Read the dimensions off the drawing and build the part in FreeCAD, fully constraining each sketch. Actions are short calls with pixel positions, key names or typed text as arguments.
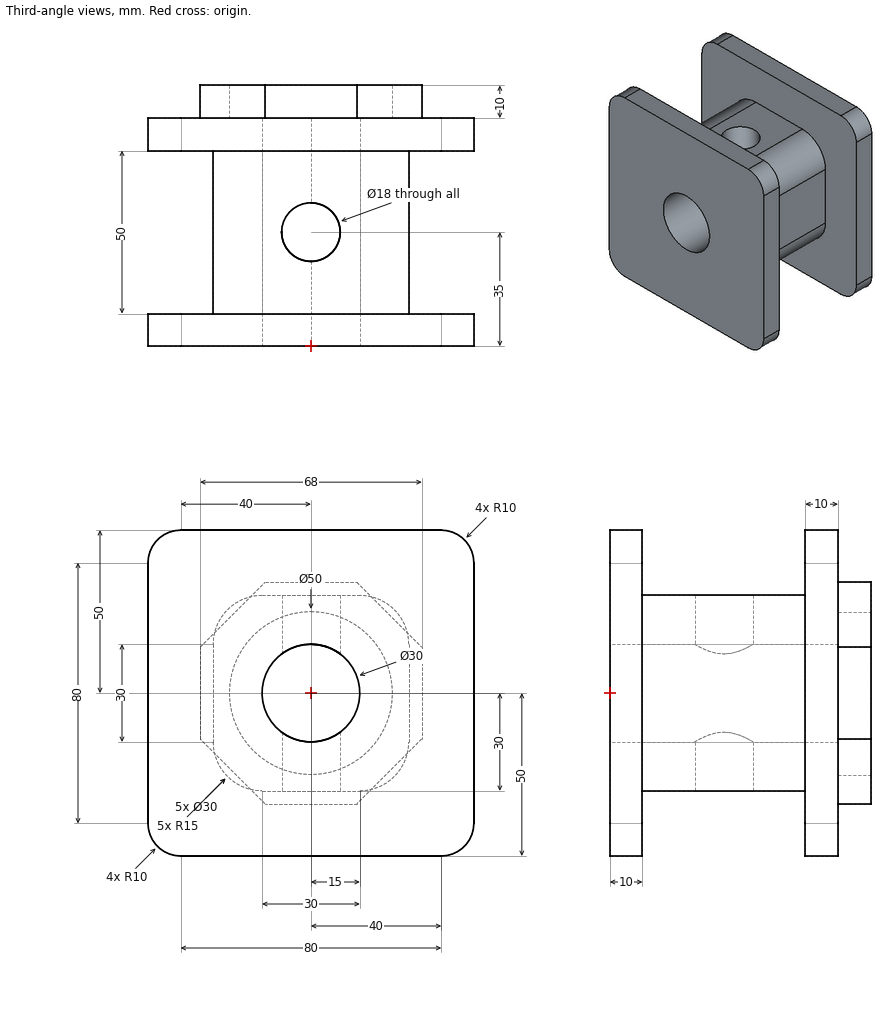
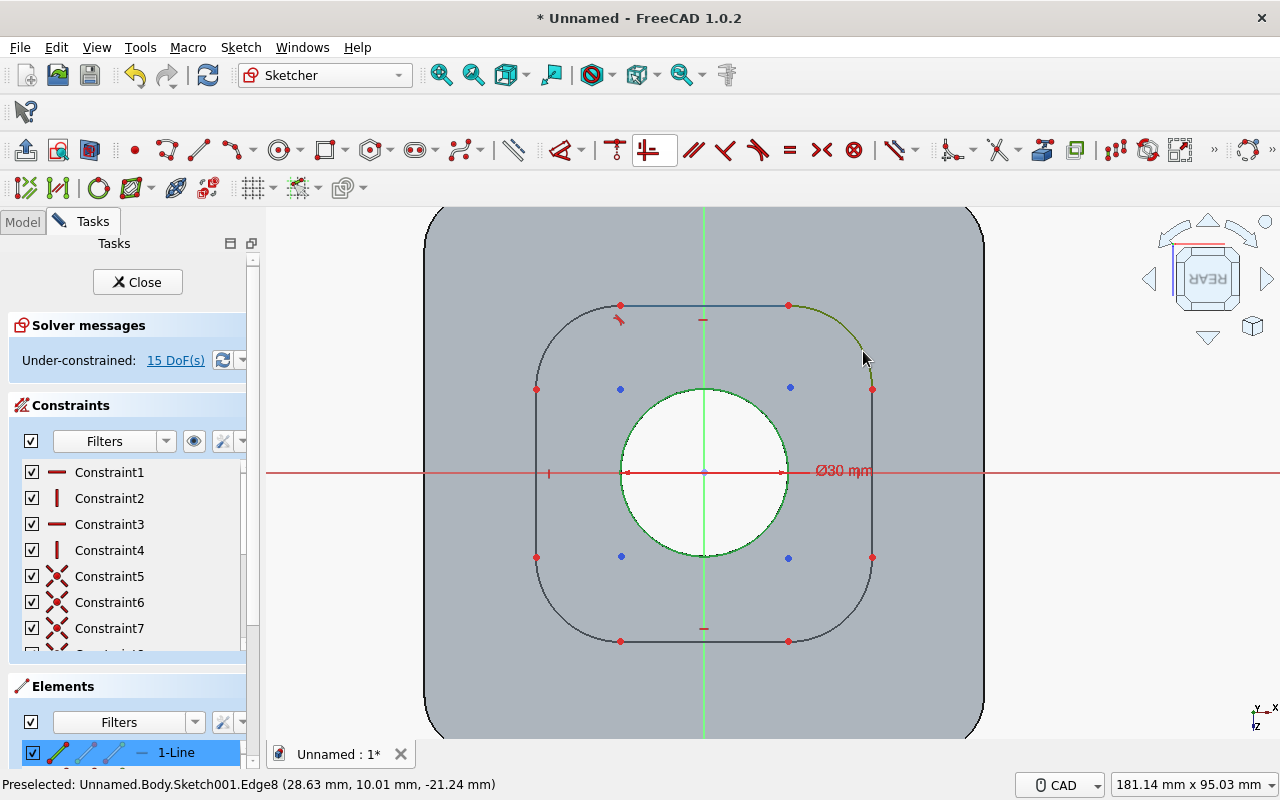
click(758, 150)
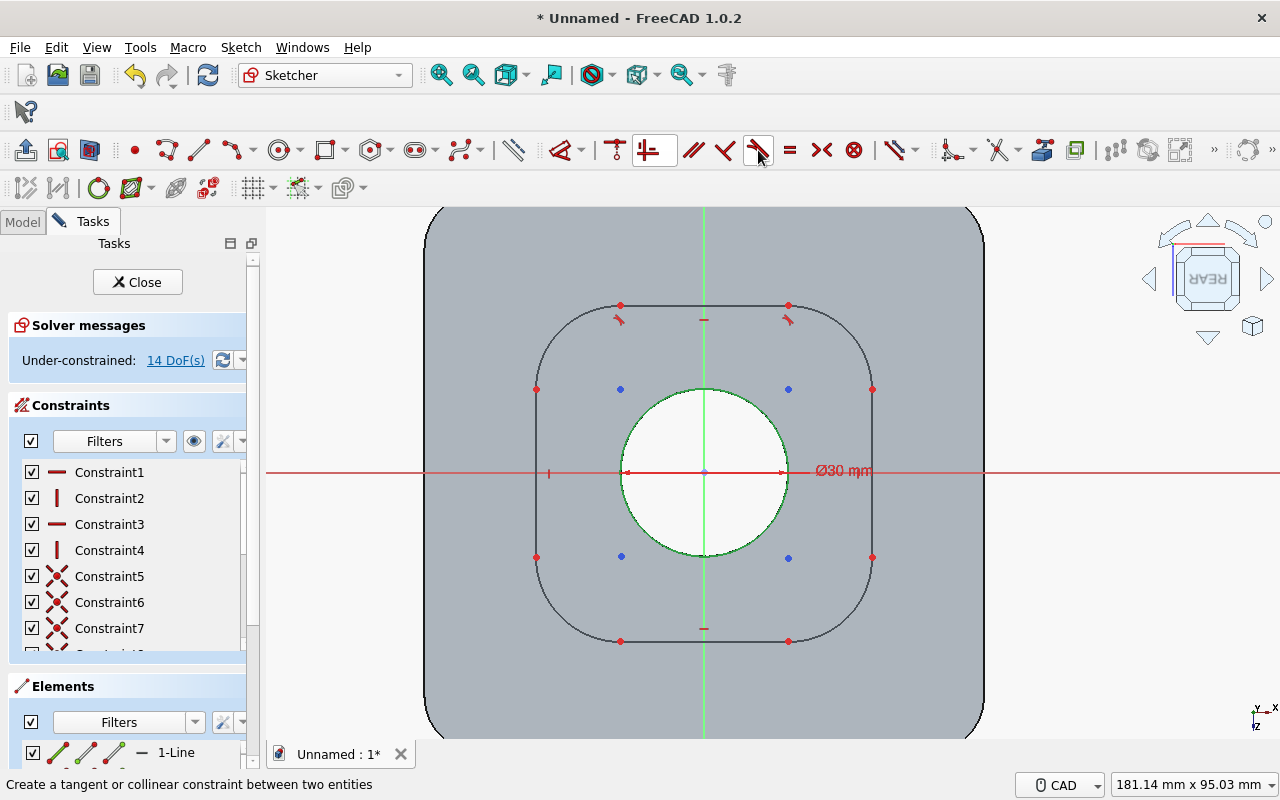
click(536, 440)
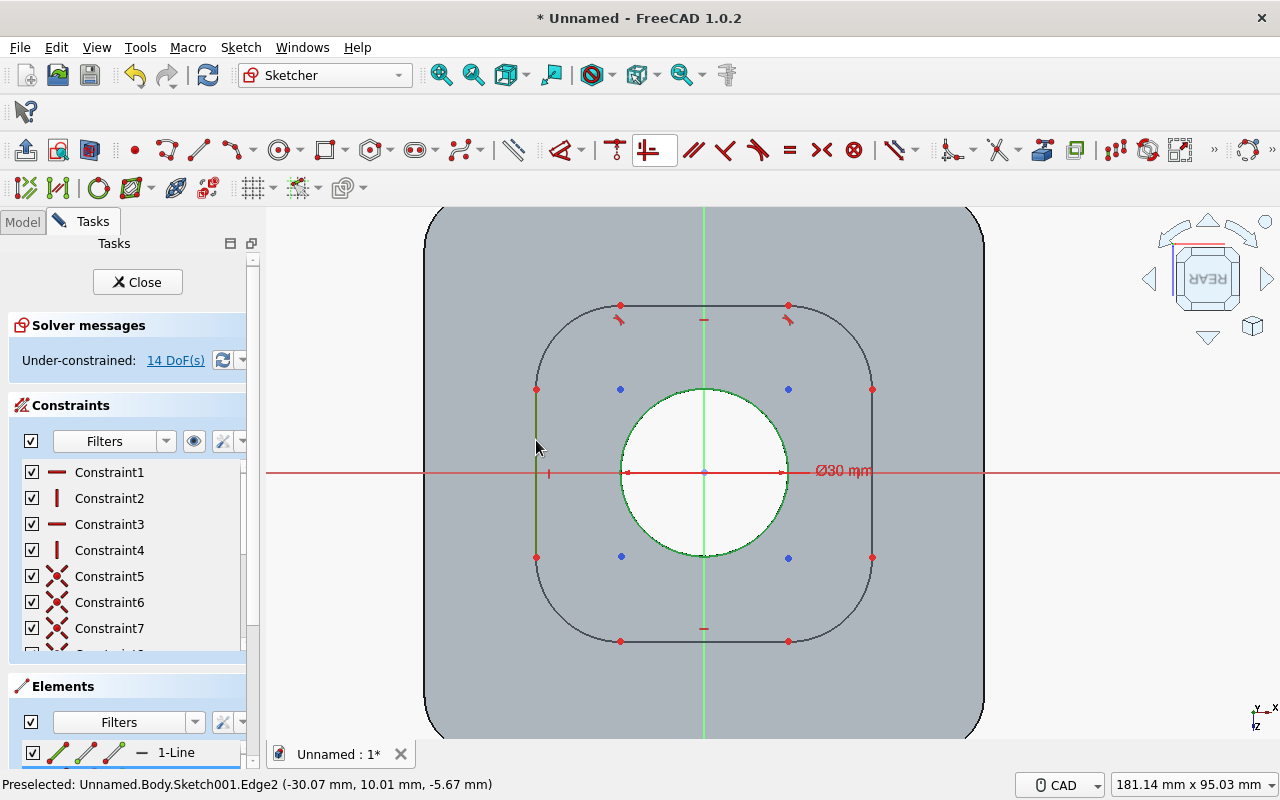
click(582, 315)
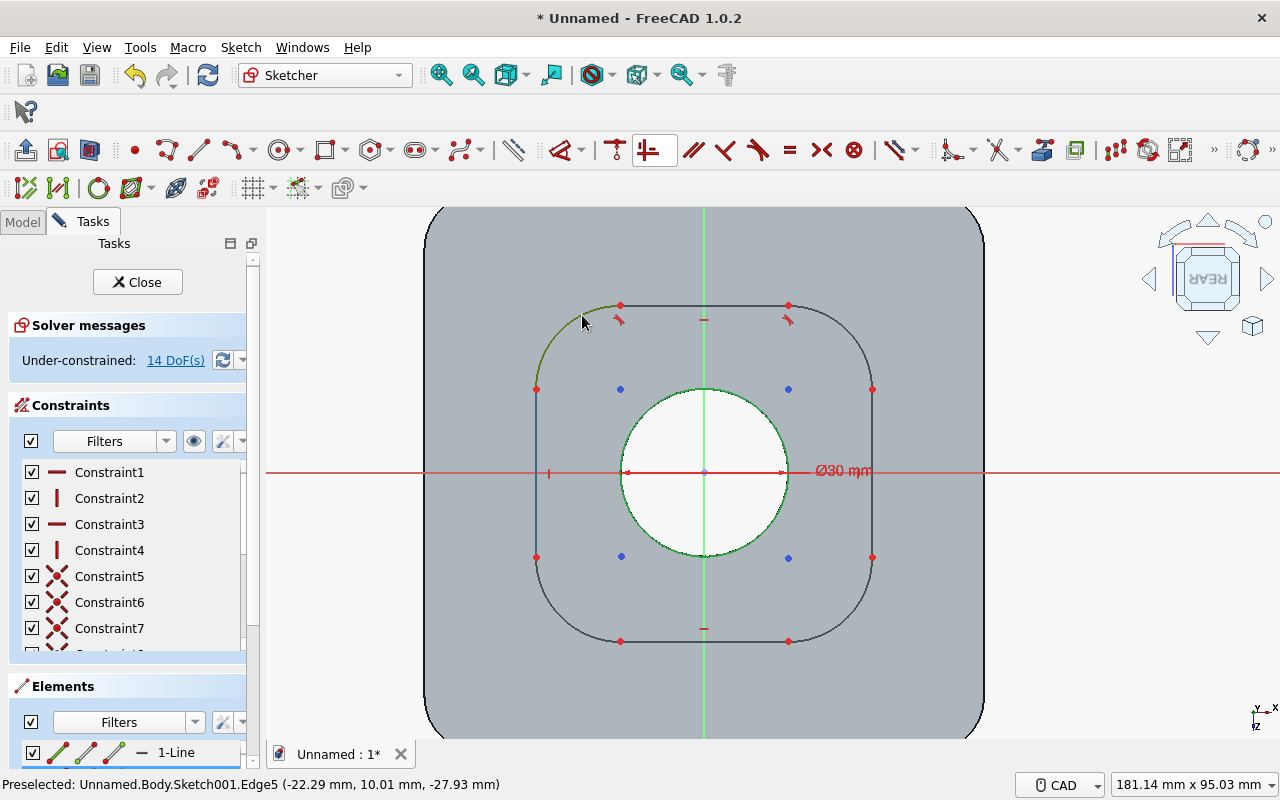
click(758, 150)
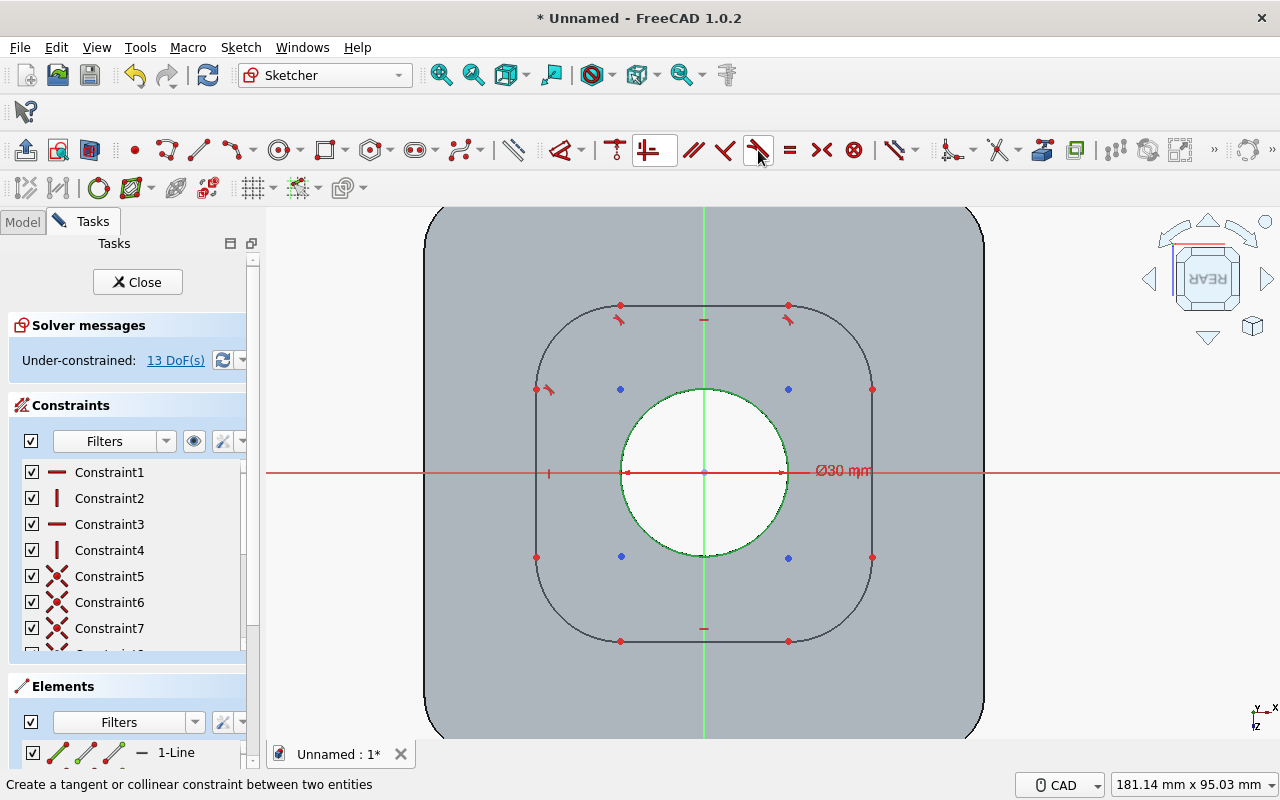
click(536, 440)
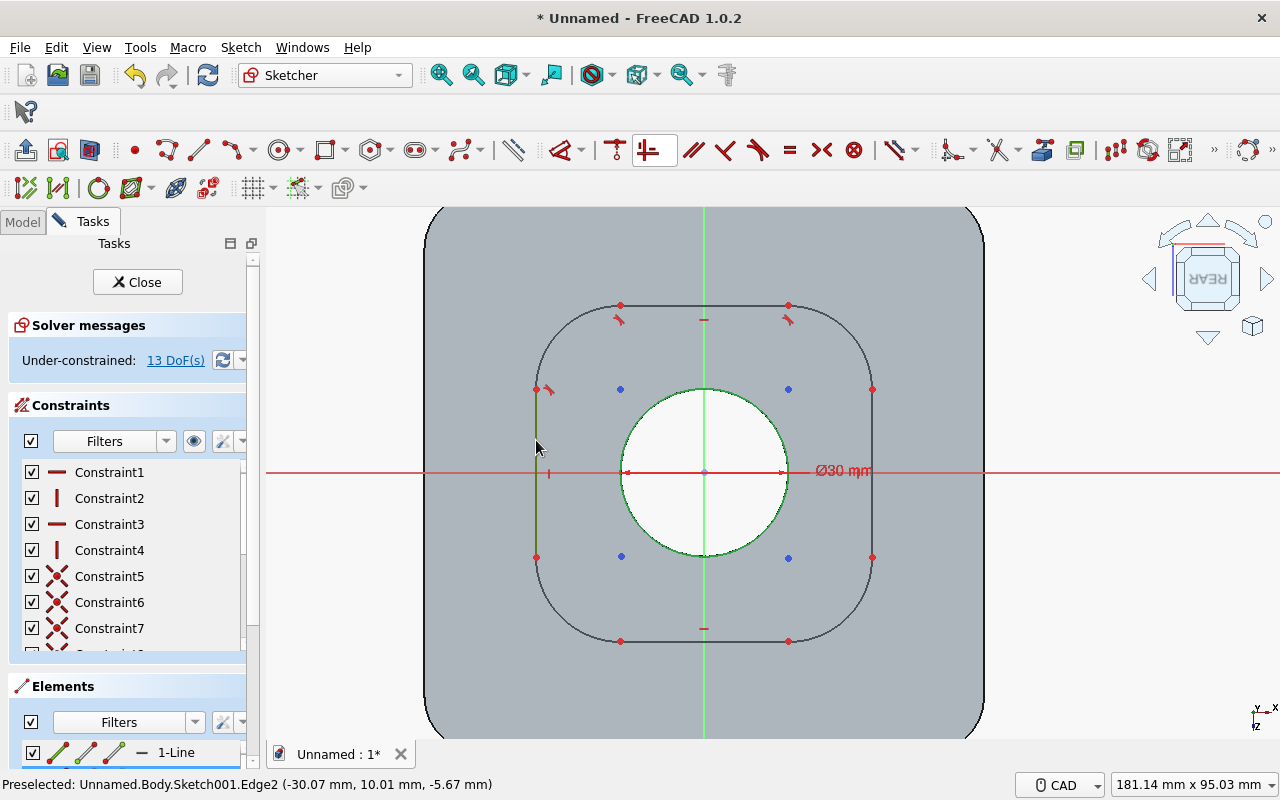
click(546, 596)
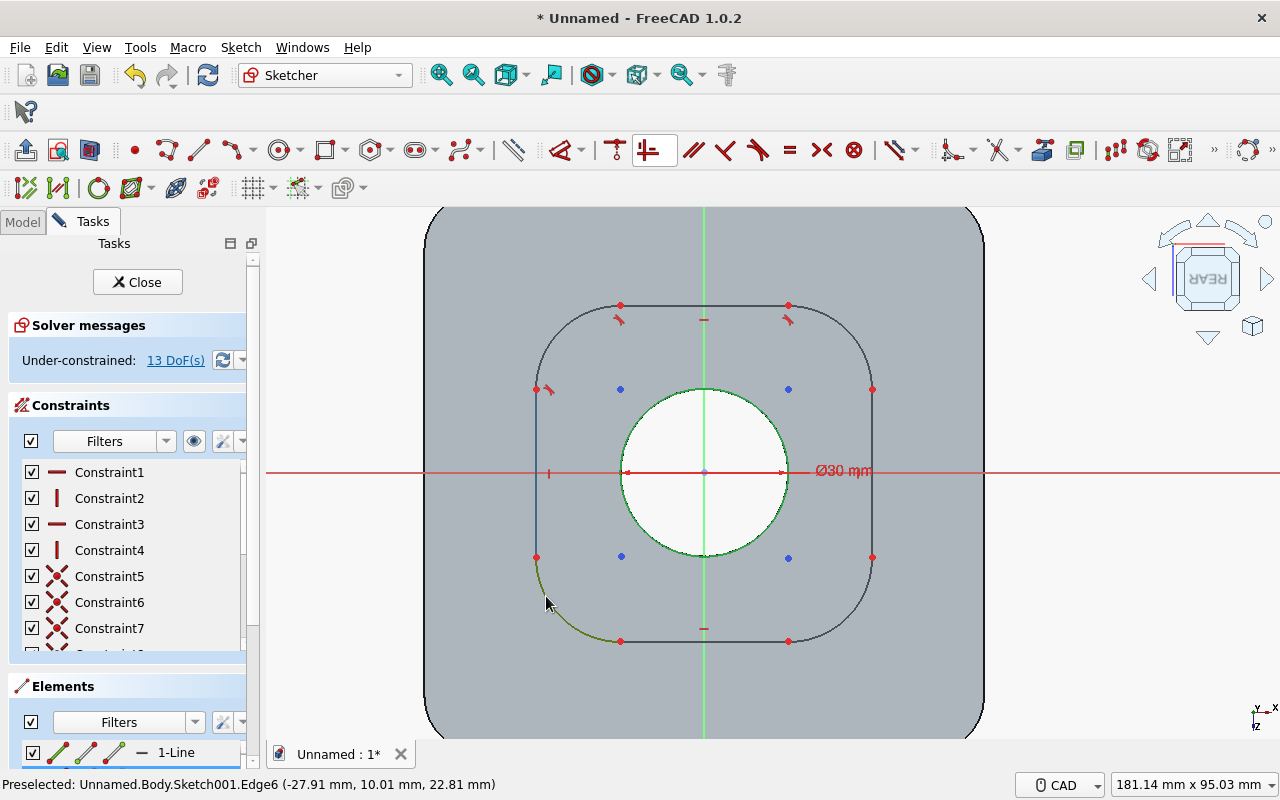
click(758, 150)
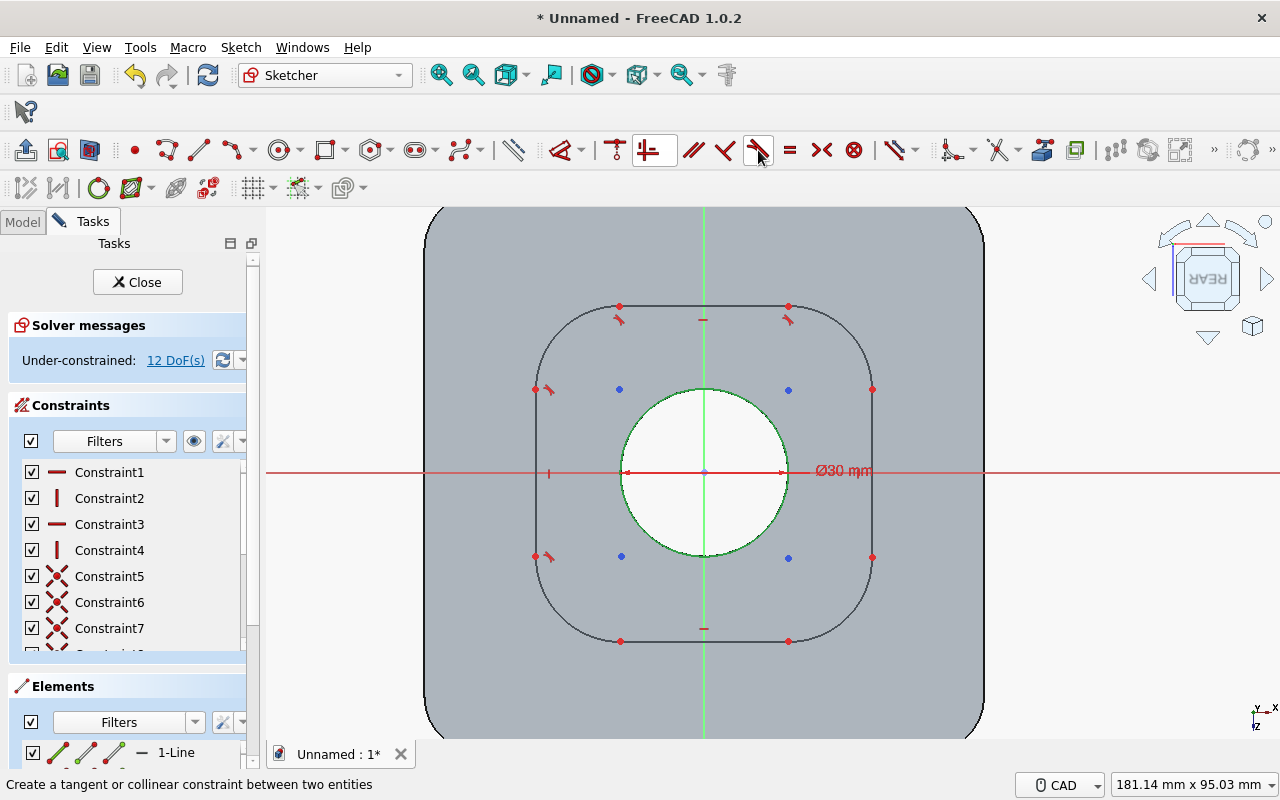
click(670, 642)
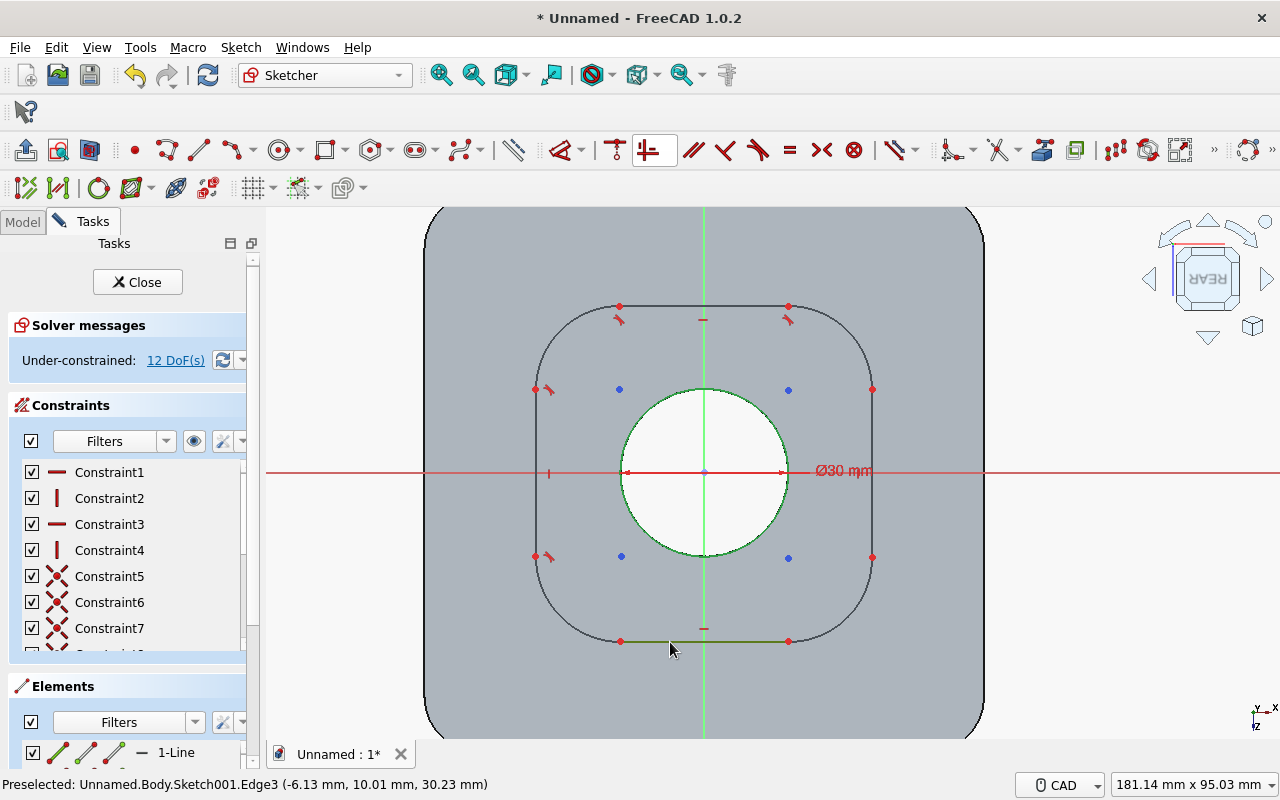
click(545, 595)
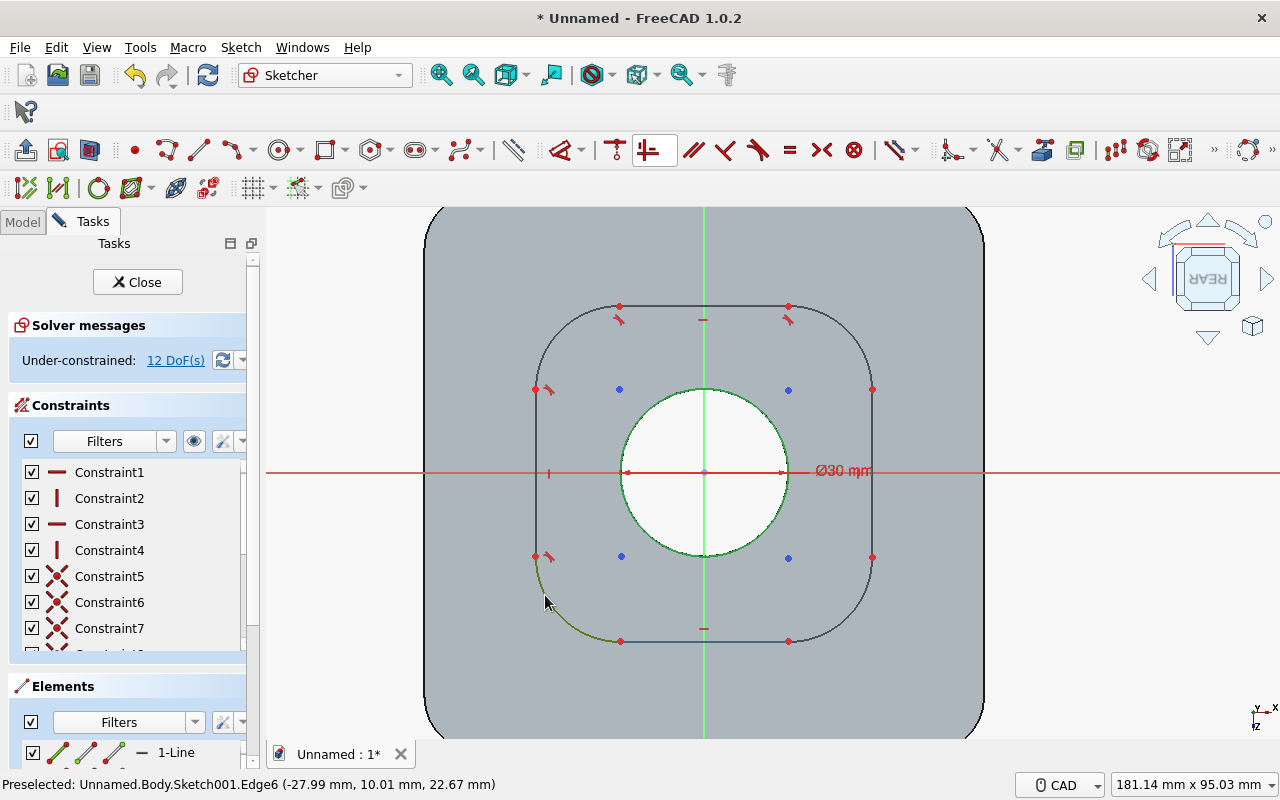
click(758, 150)